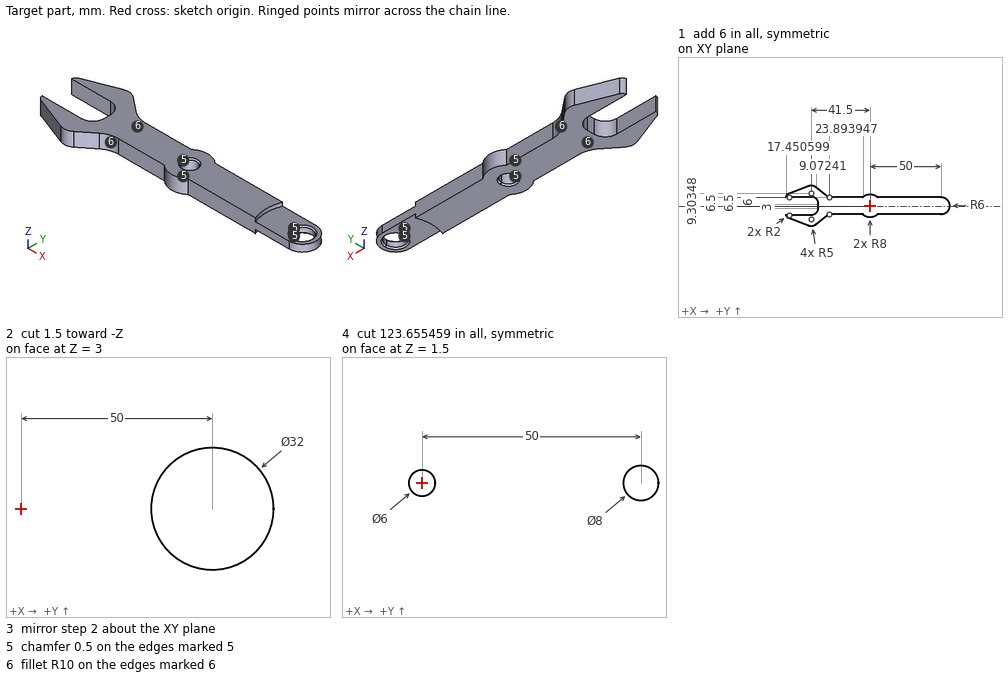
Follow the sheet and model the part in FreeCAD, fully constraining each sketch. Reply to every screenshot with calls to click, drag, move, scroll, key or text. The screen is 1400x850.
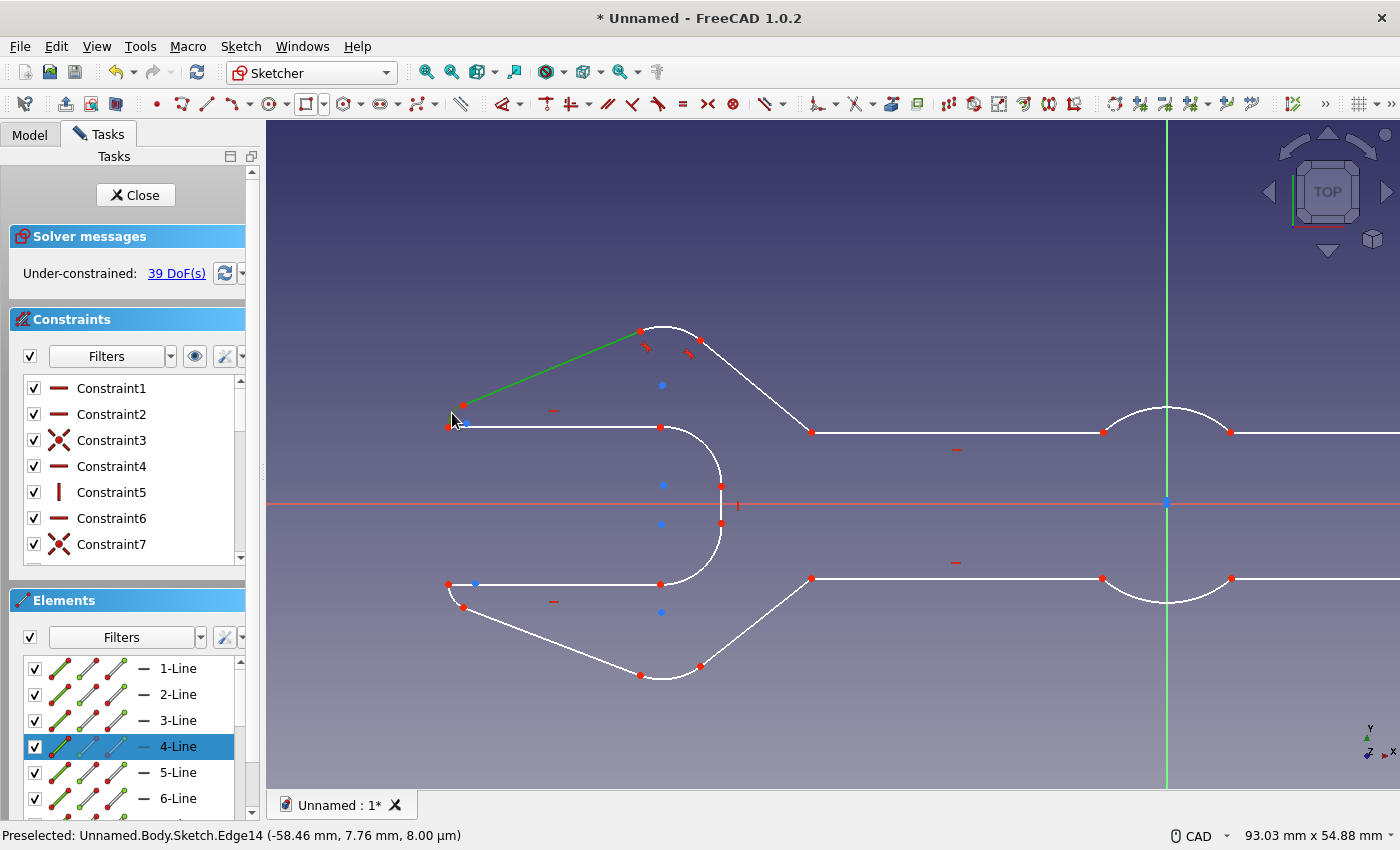
click(658, 104)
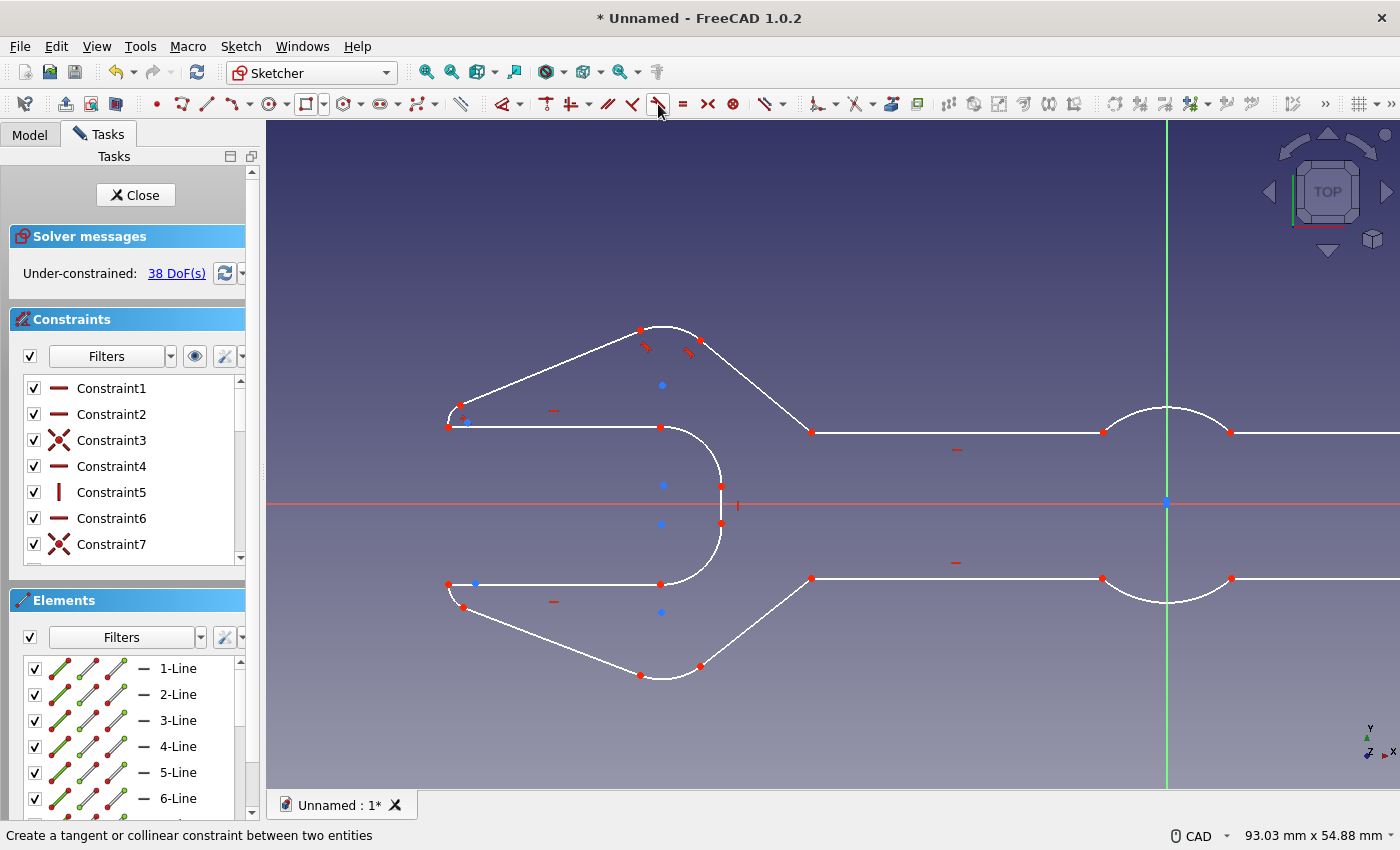
click(512, 427)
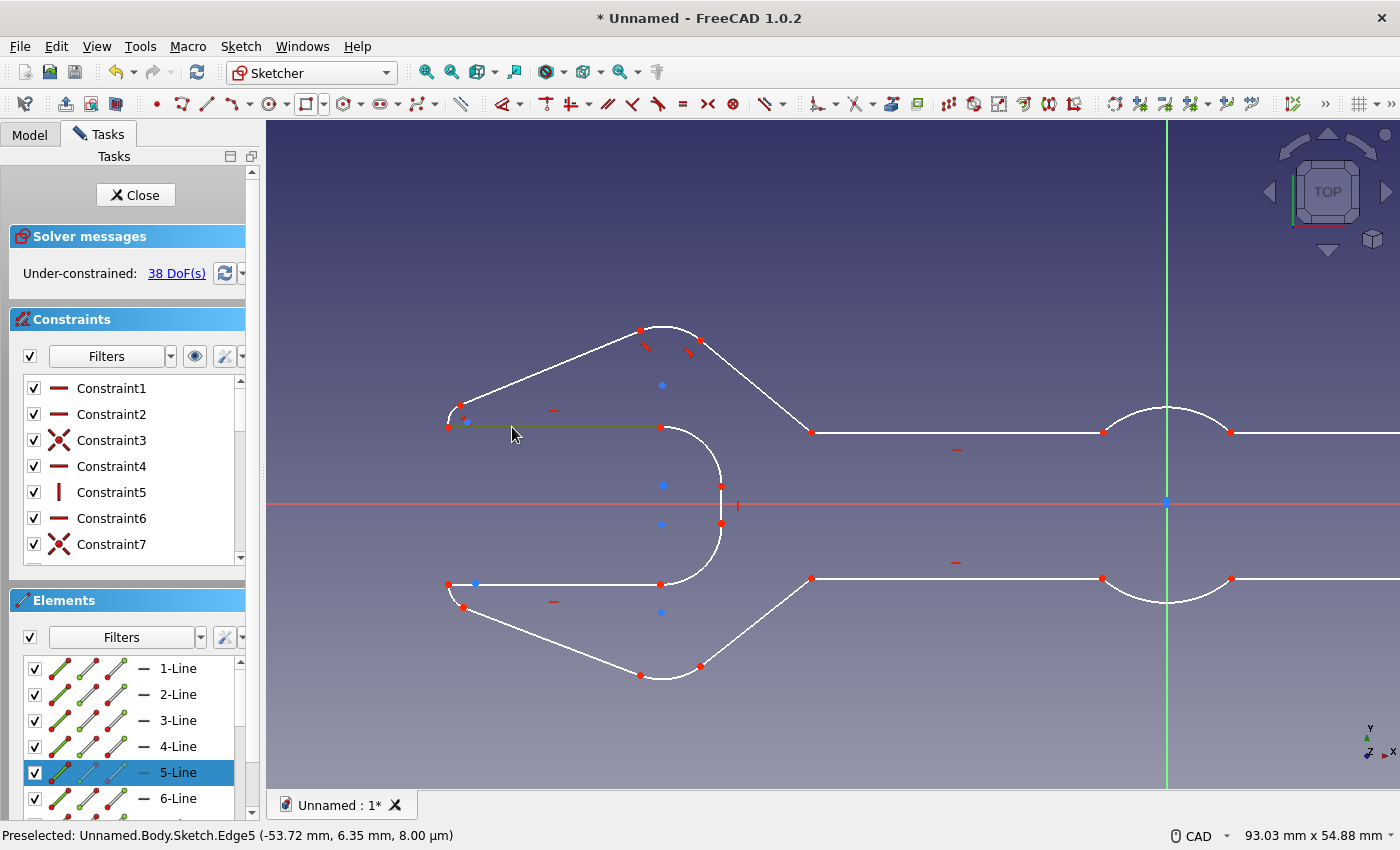
click(715, 459)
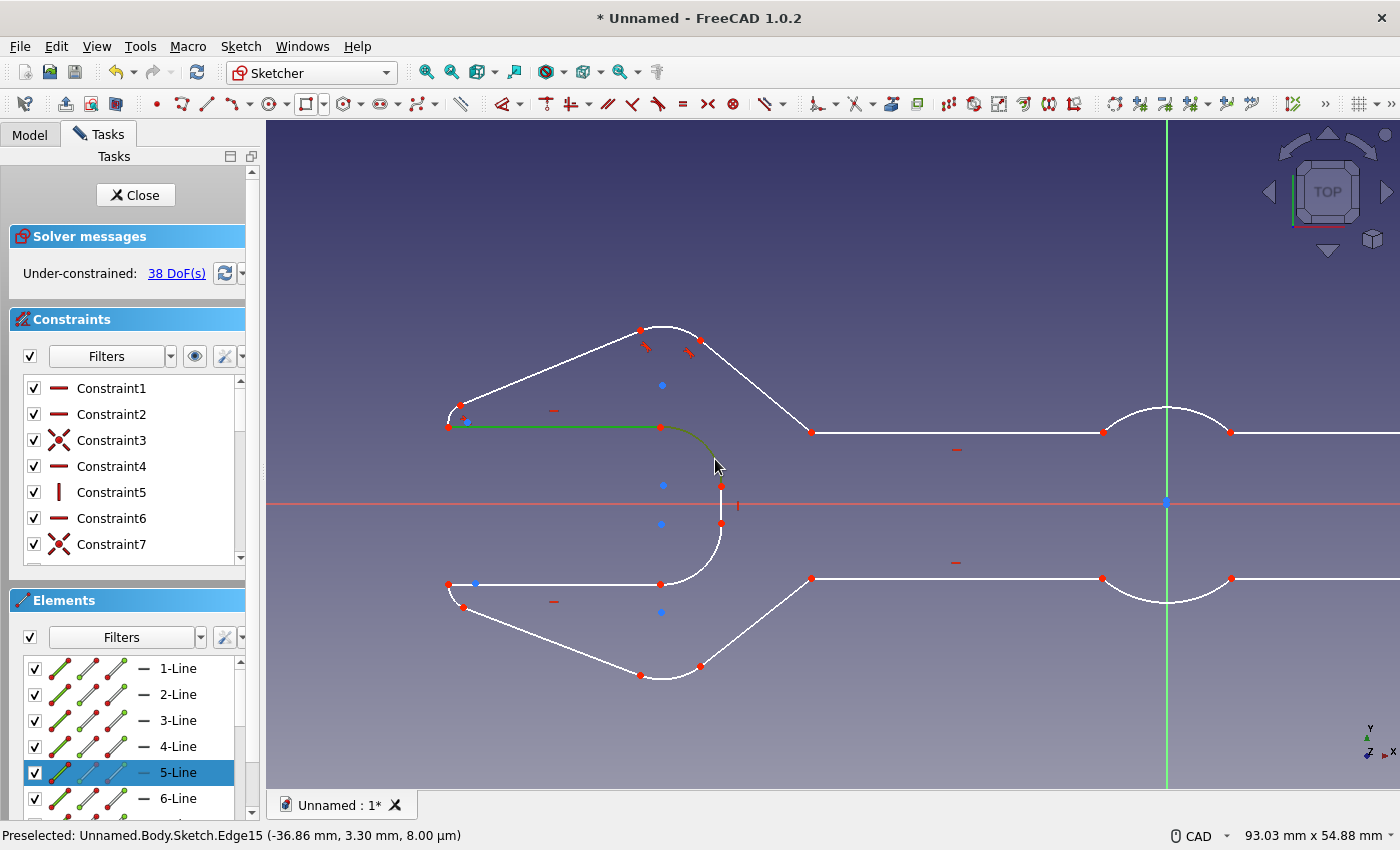
click(658, 104)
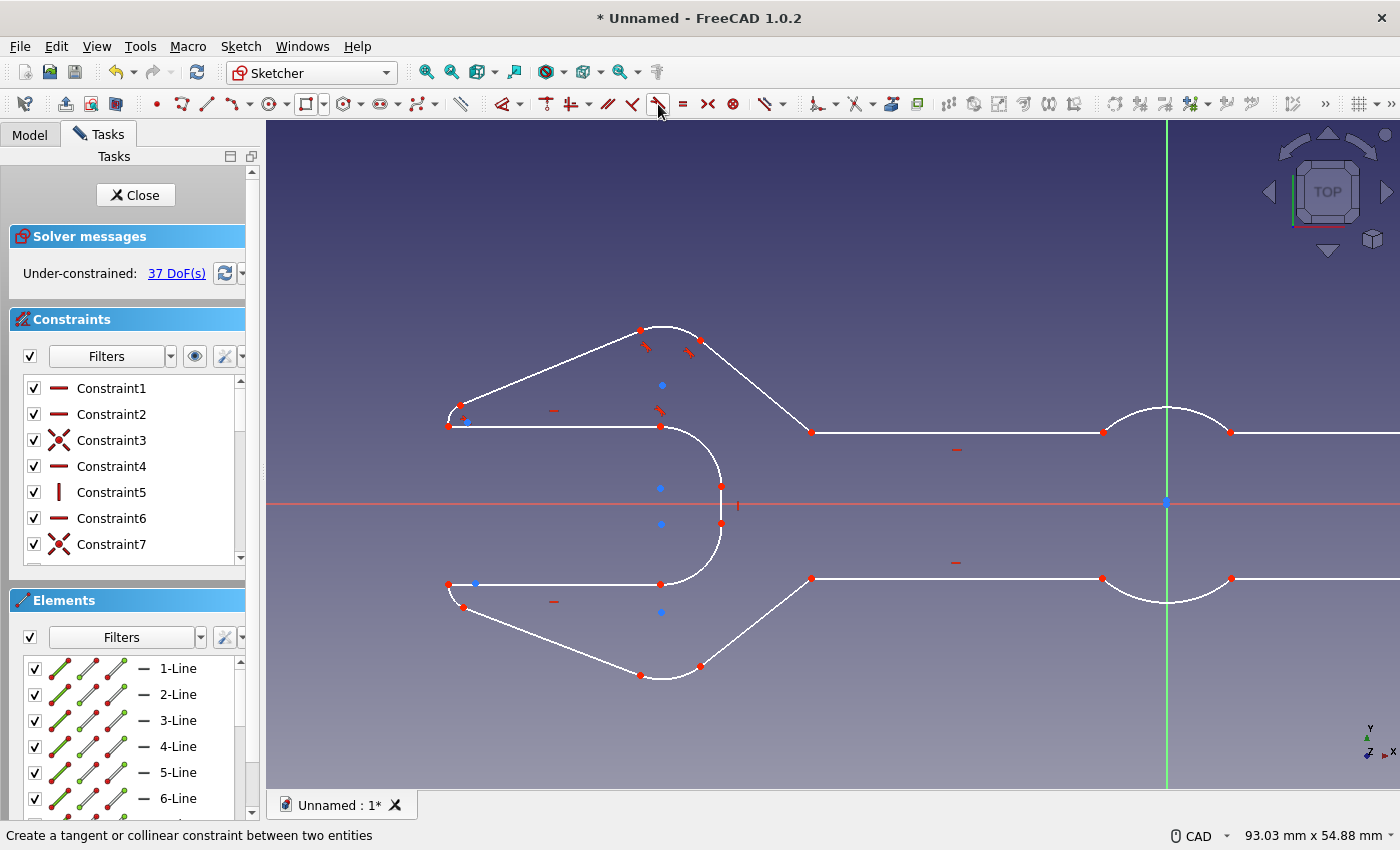
click(721, 502)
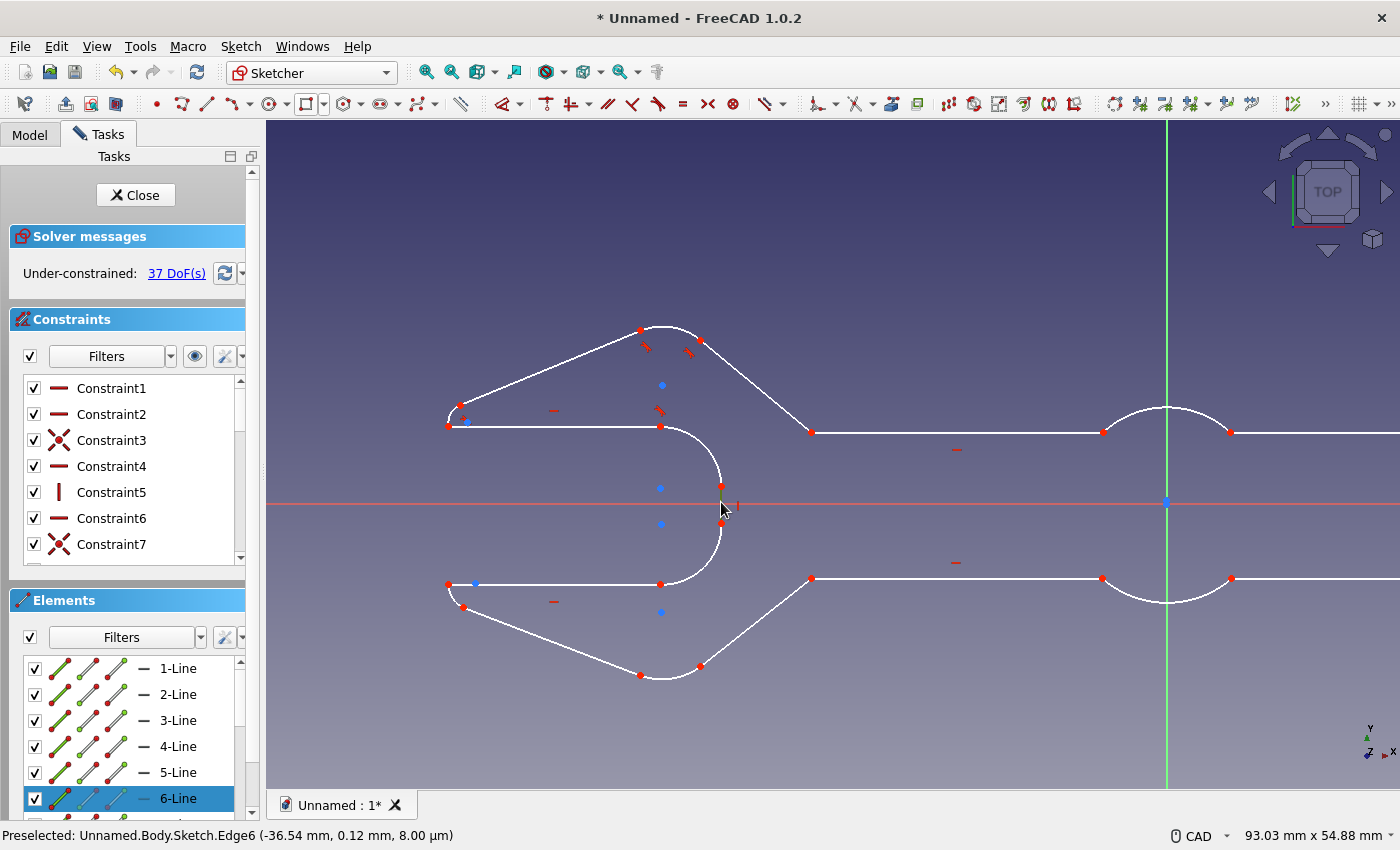
click(714, 460)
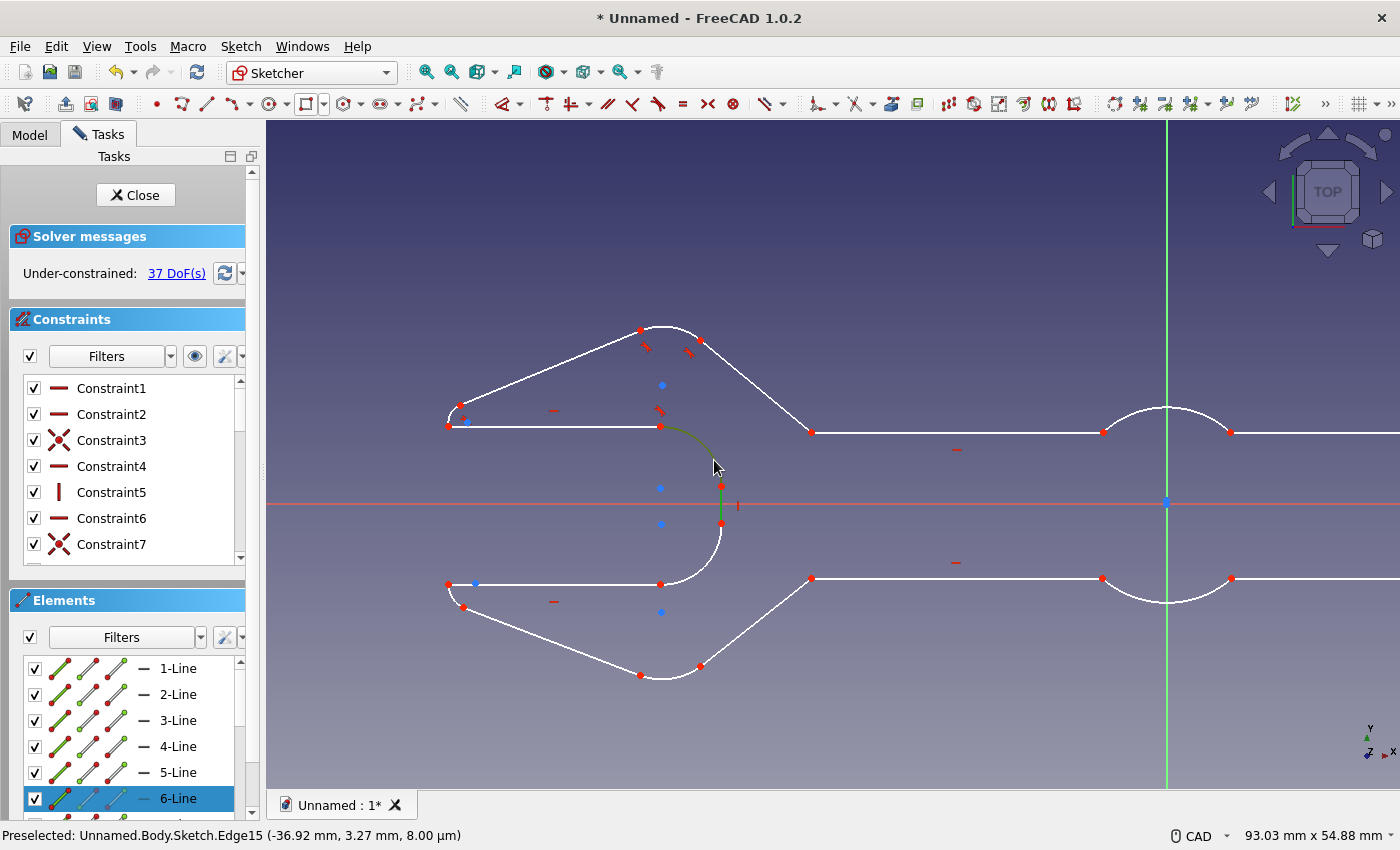
click(658, 104)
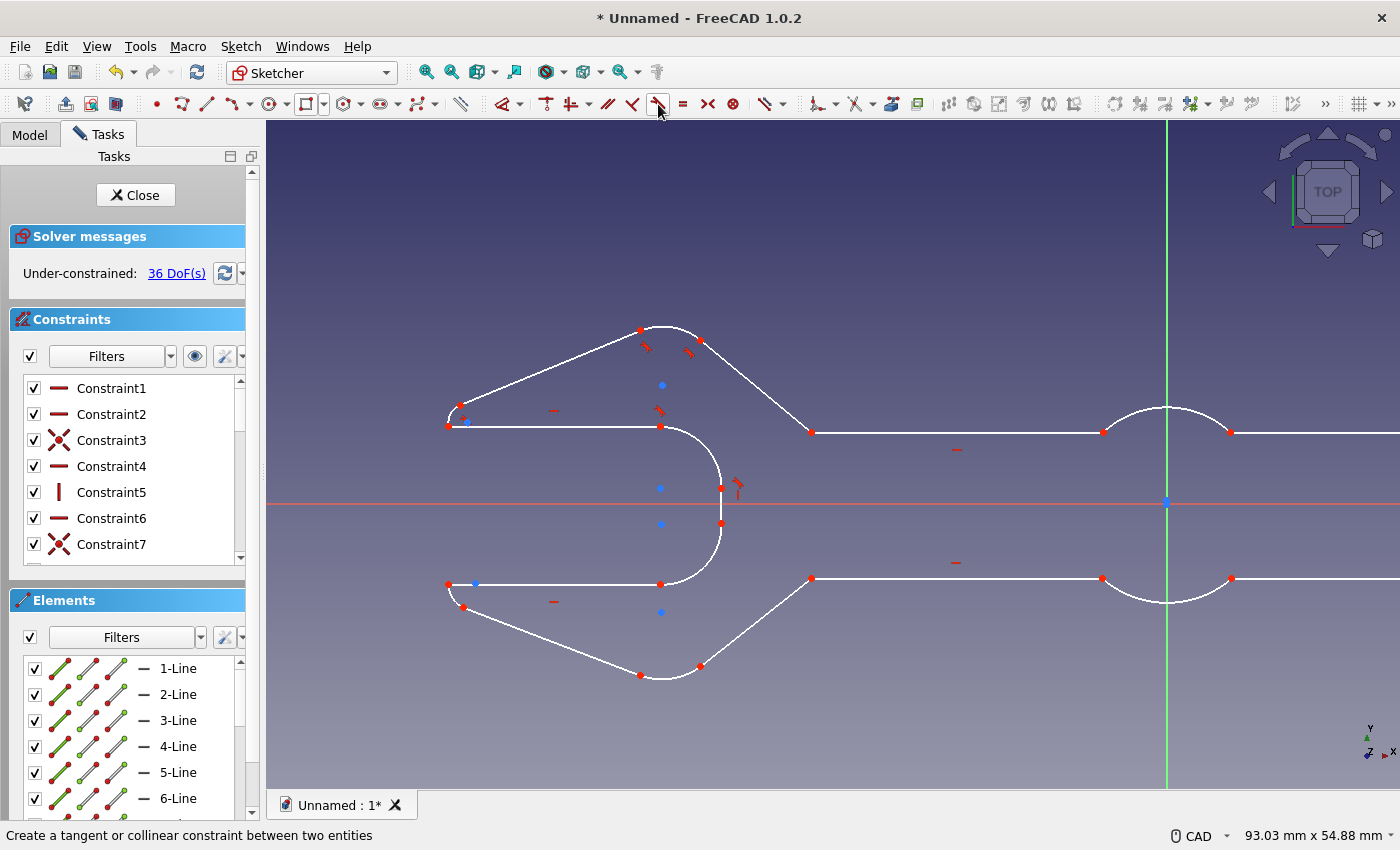
click(721, 502)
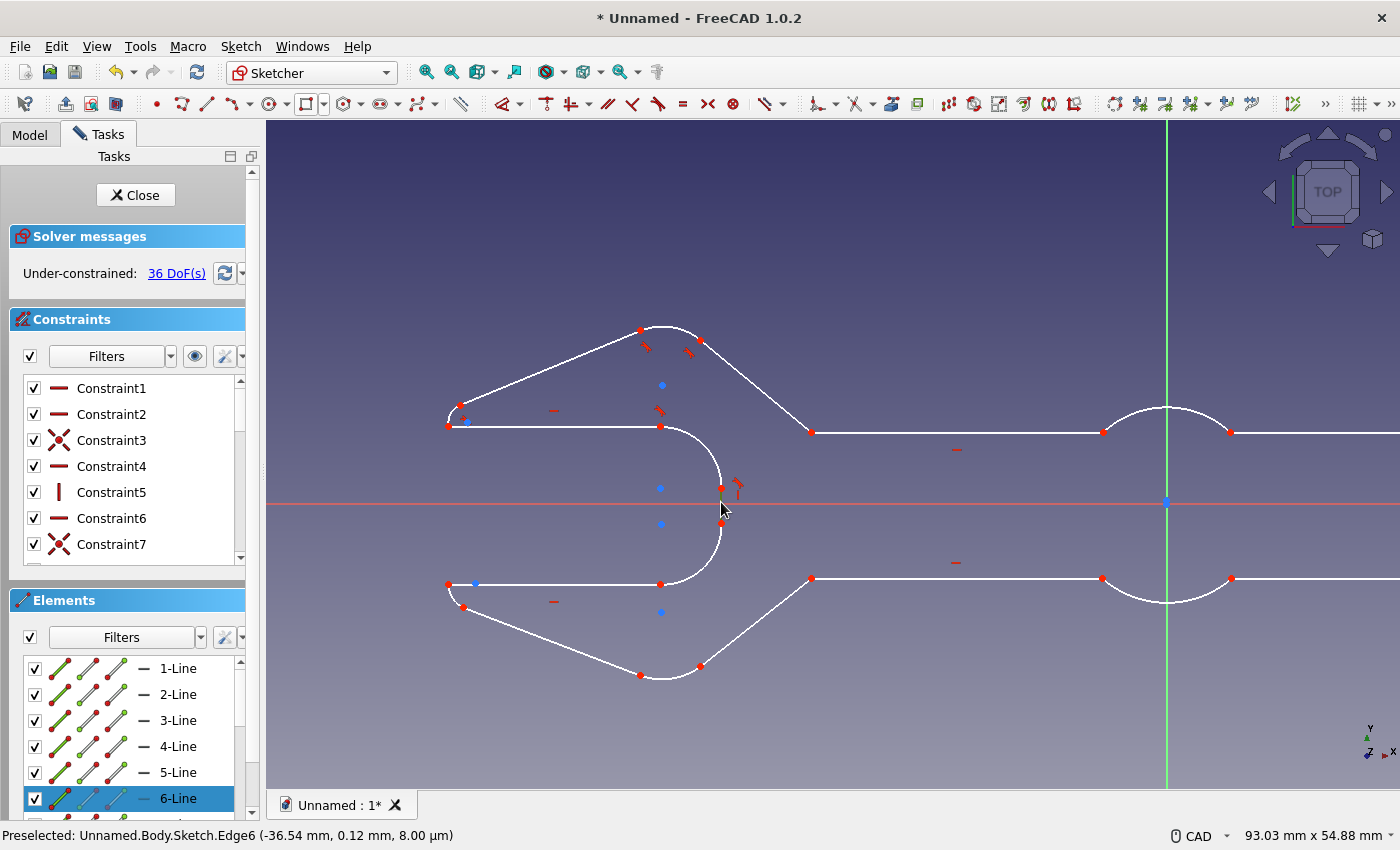
click(688, 578)